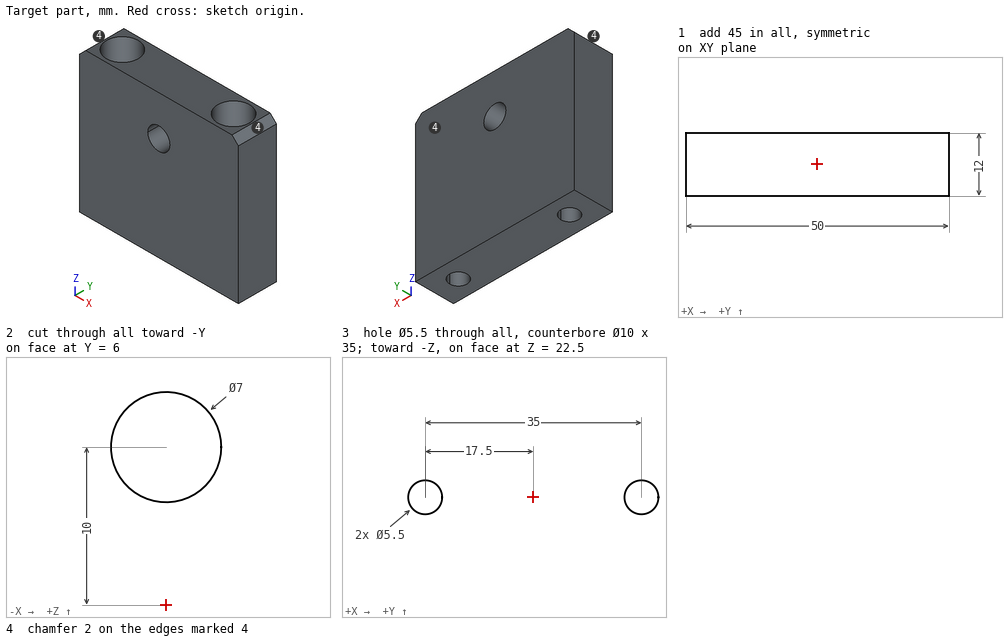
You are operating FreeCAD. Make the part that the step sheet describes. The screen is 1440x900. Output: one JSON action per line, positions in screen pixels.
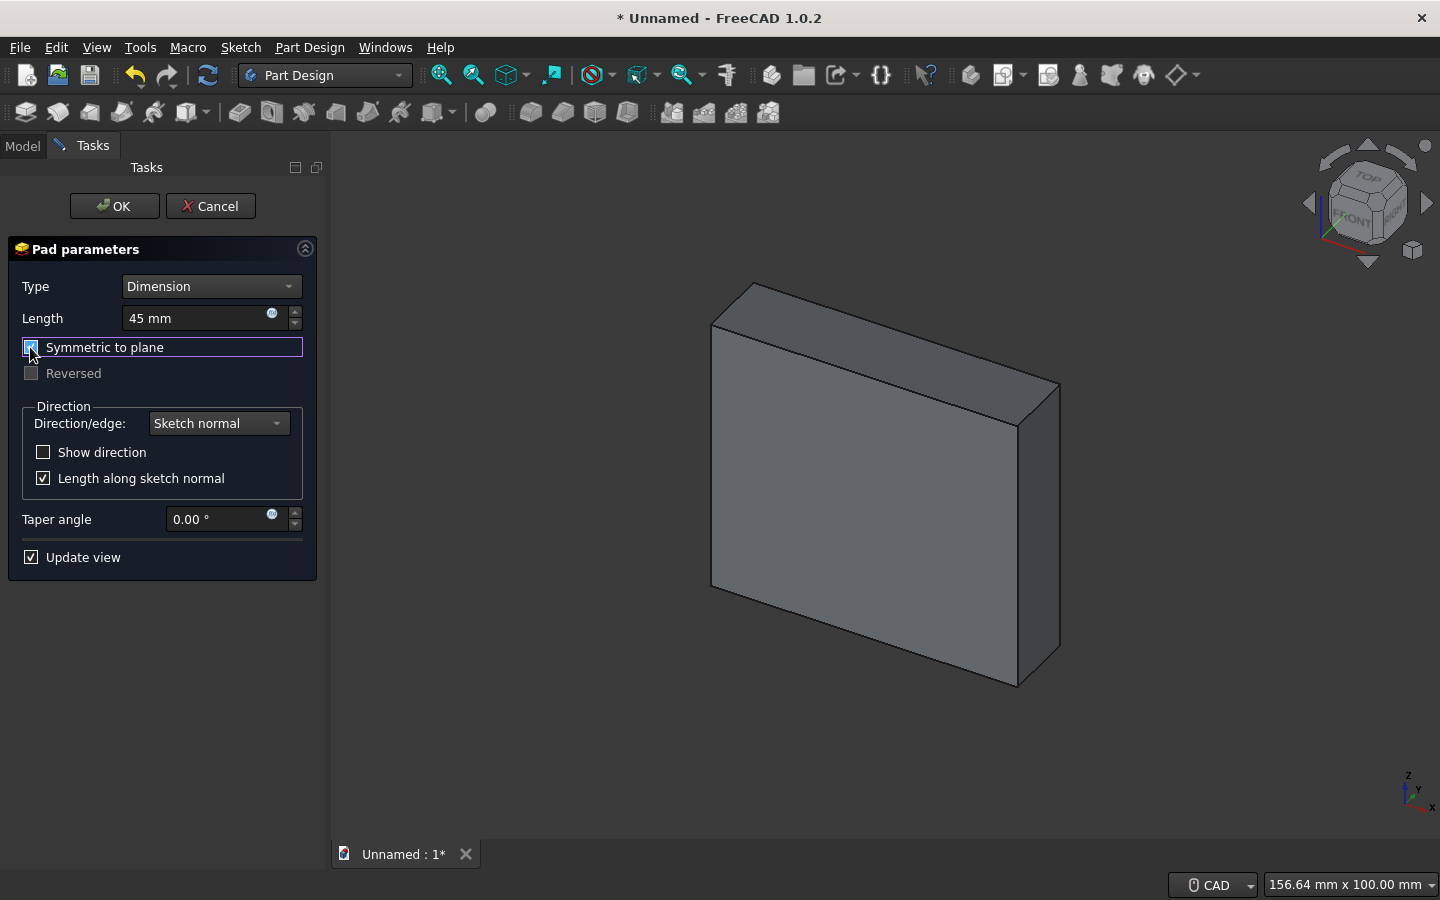
{"action": "left_click", "coordinate": [115, 206]}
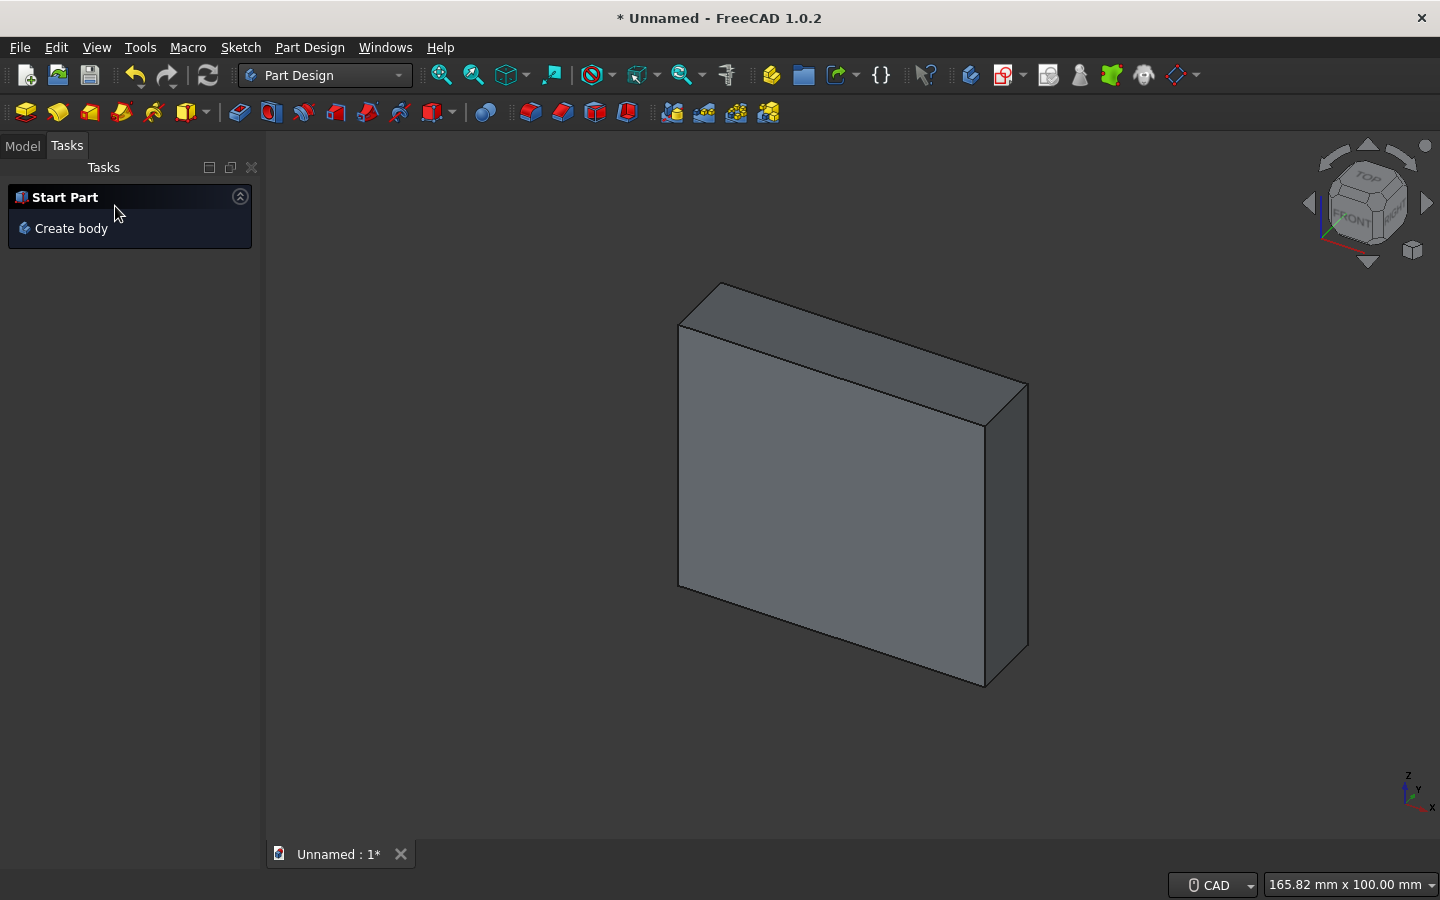
{"action": "key", "text": "4"}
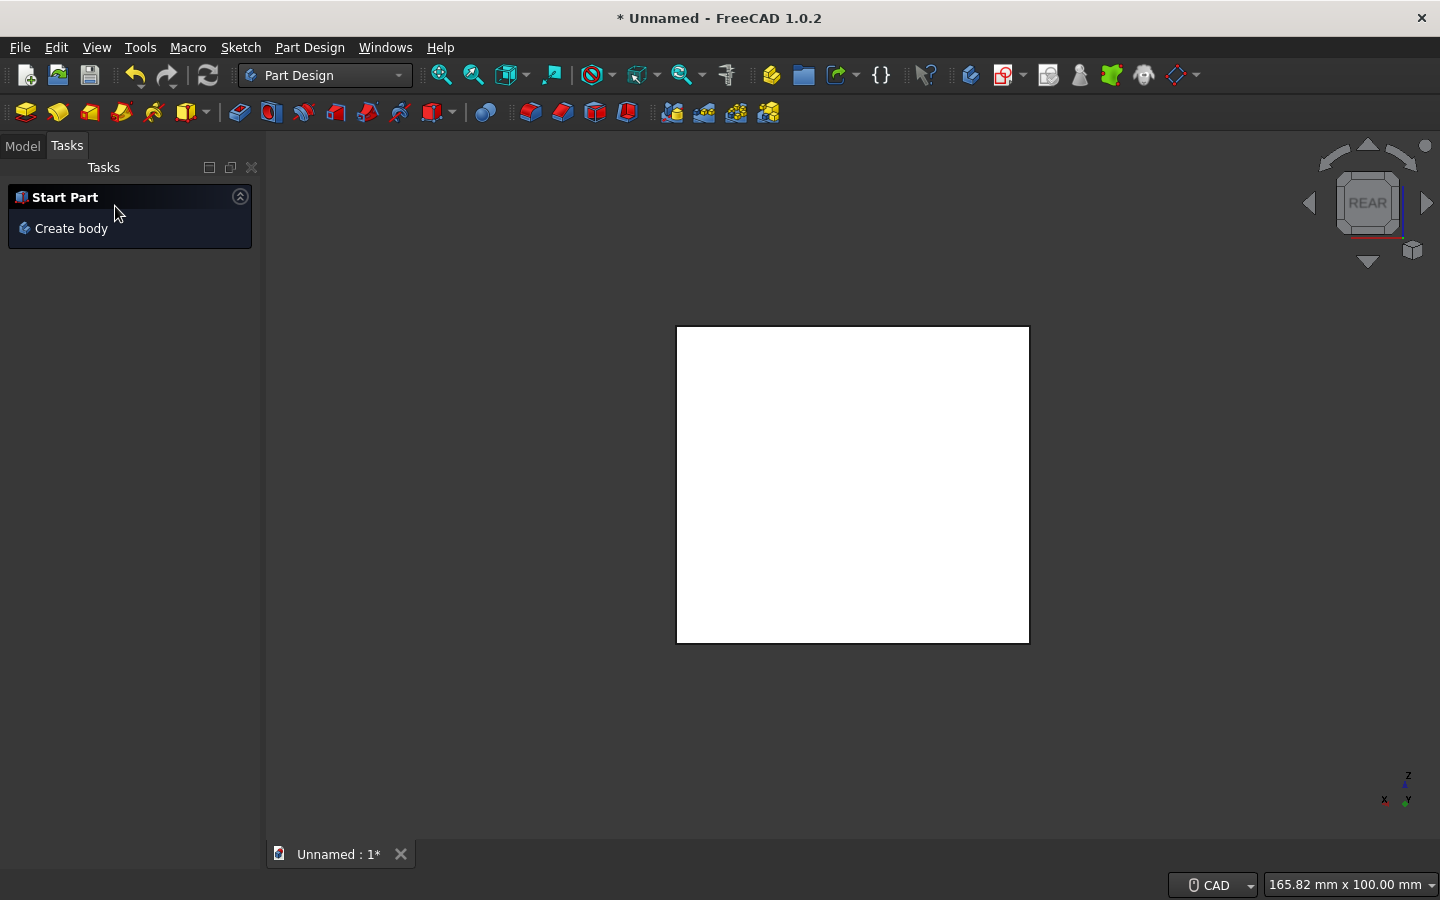
{"action": "left_click", "coordinate": [442, 76]}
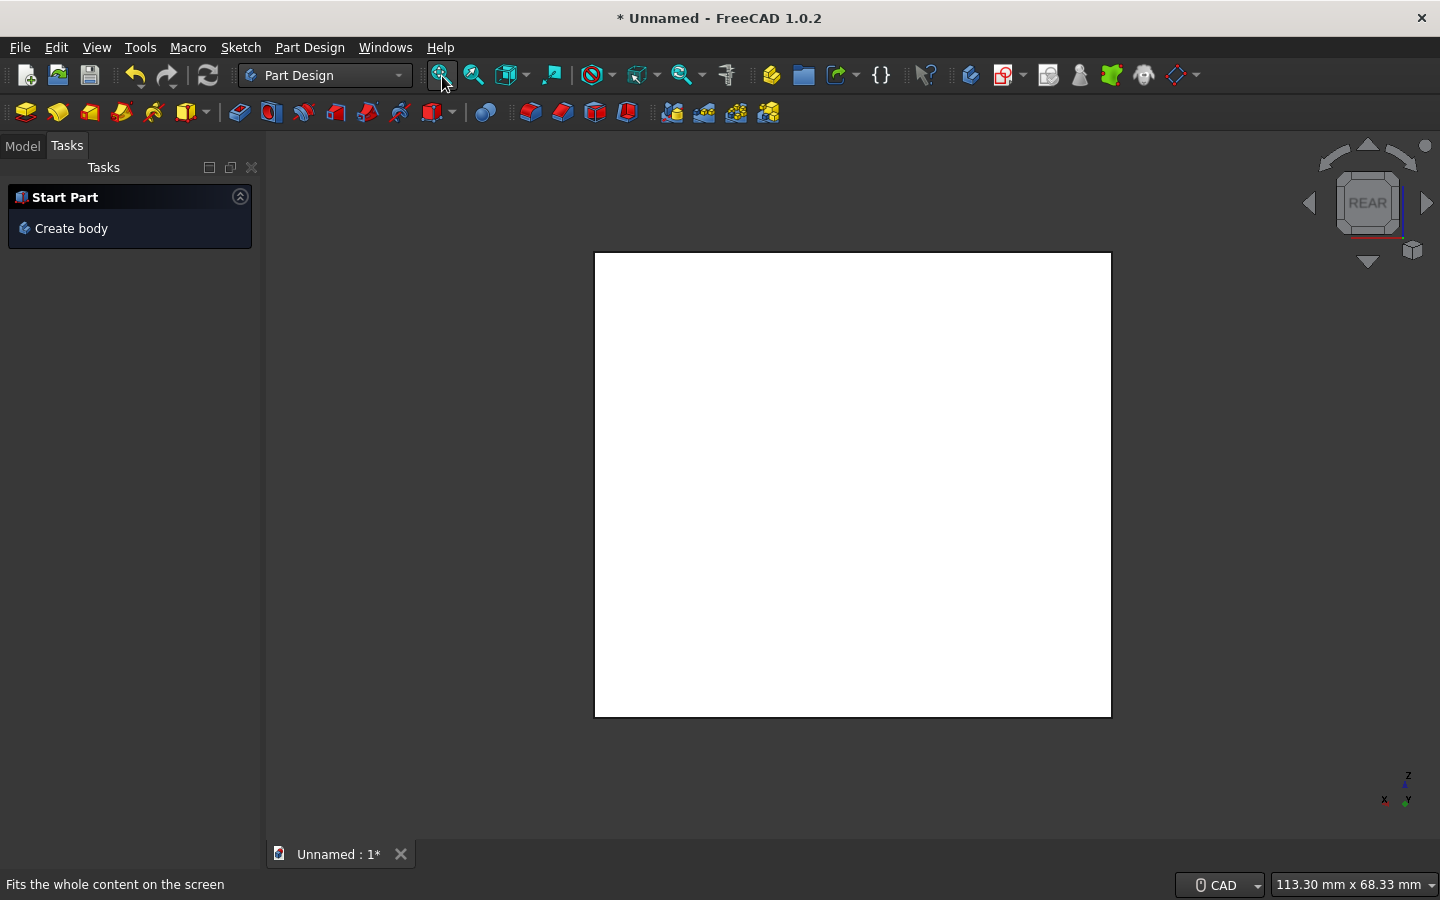
{"action": "left_click", "coordinate": [853, 484]}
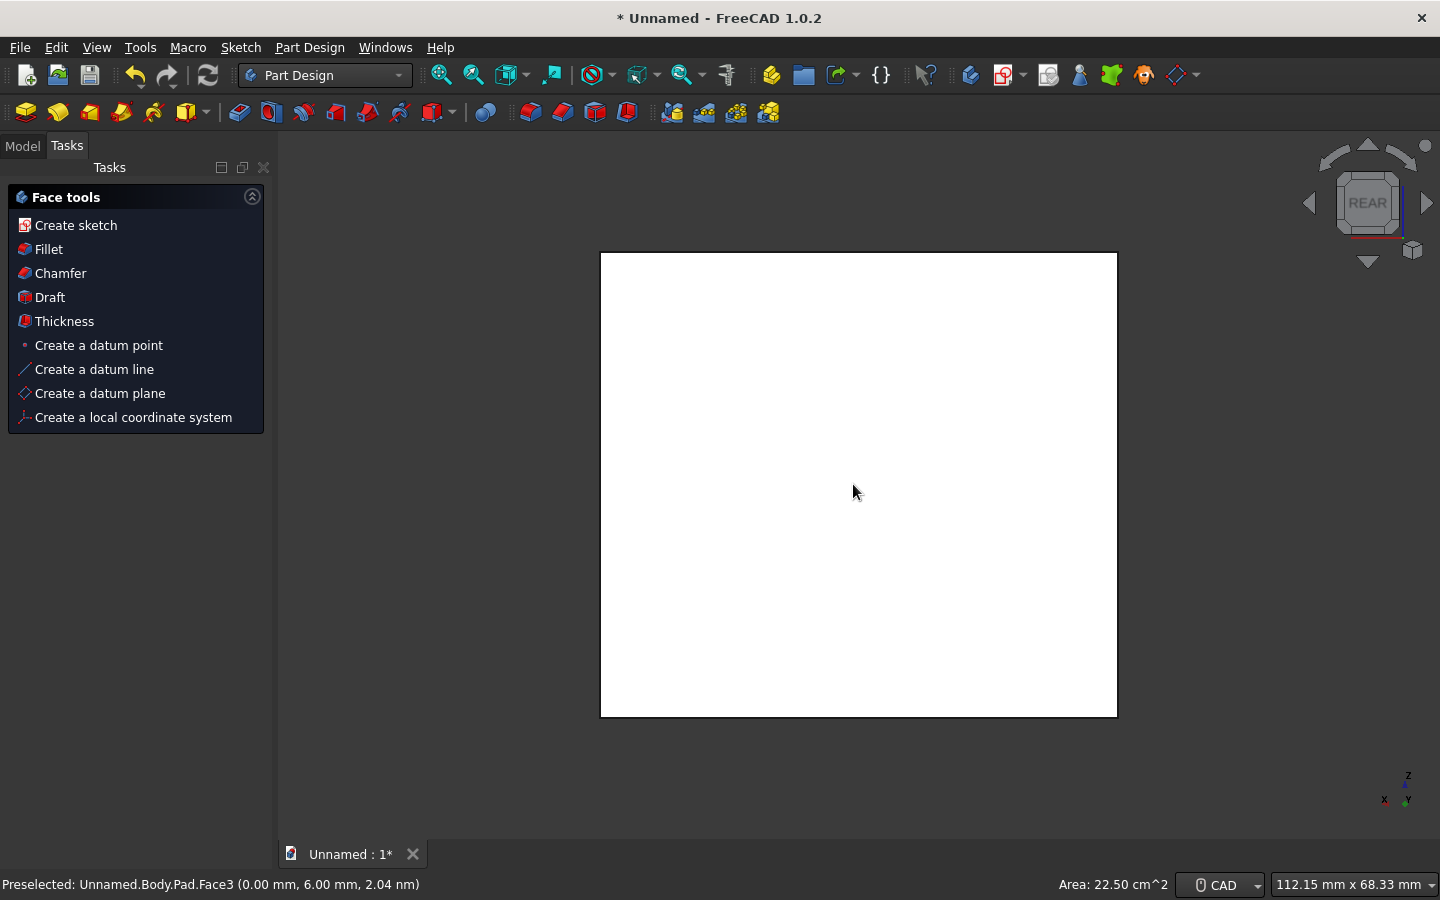
{"action": "left_click", "coordinate": [1004, 76]}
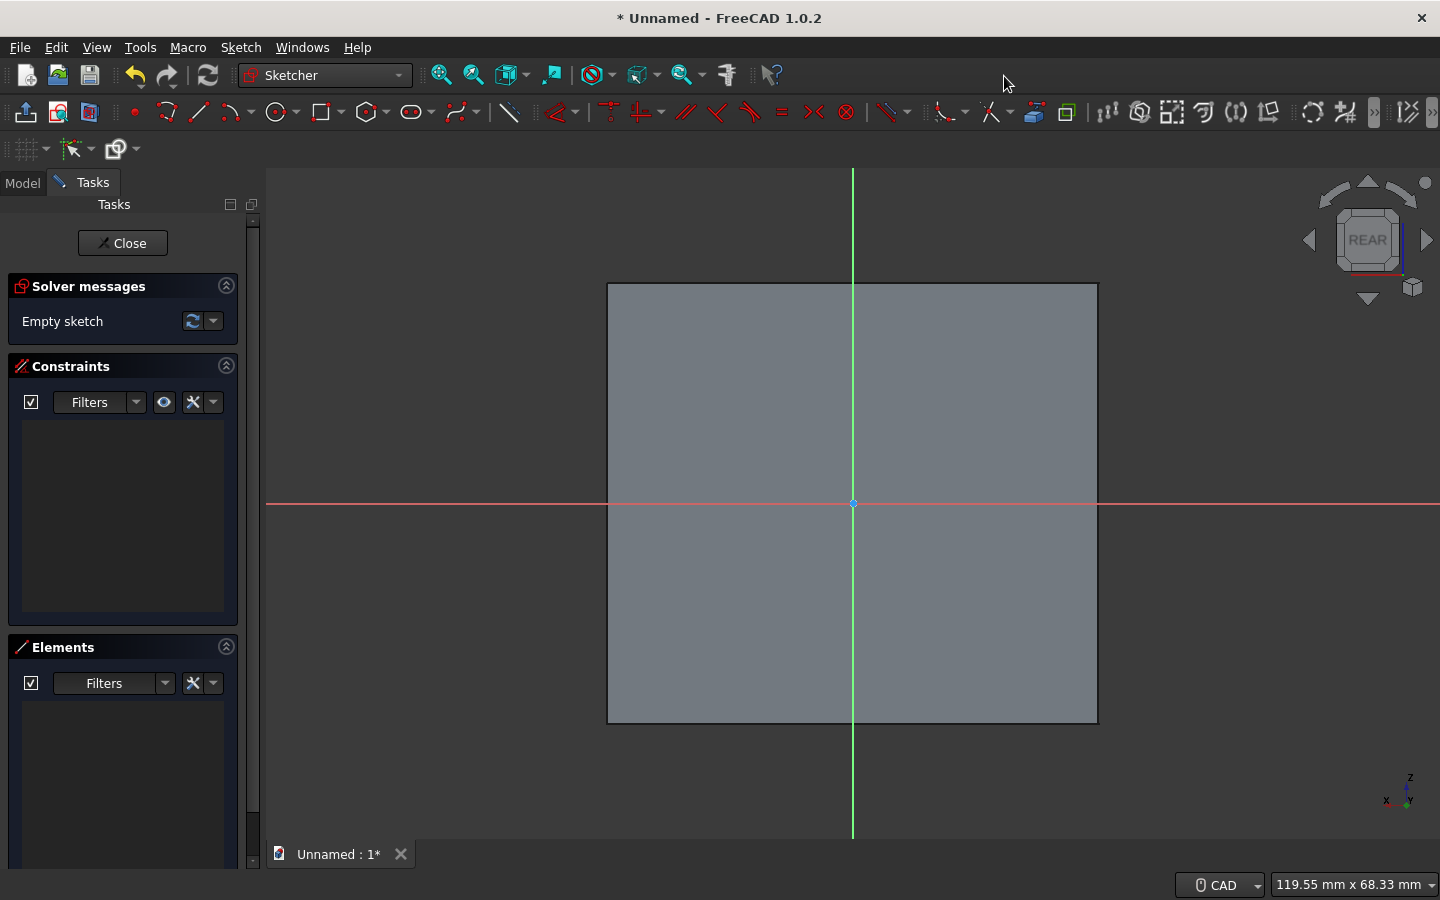
{"action": "scroll", "coordinate": [883, 409], "scroll_direction": "up", "scroll_amount": 6}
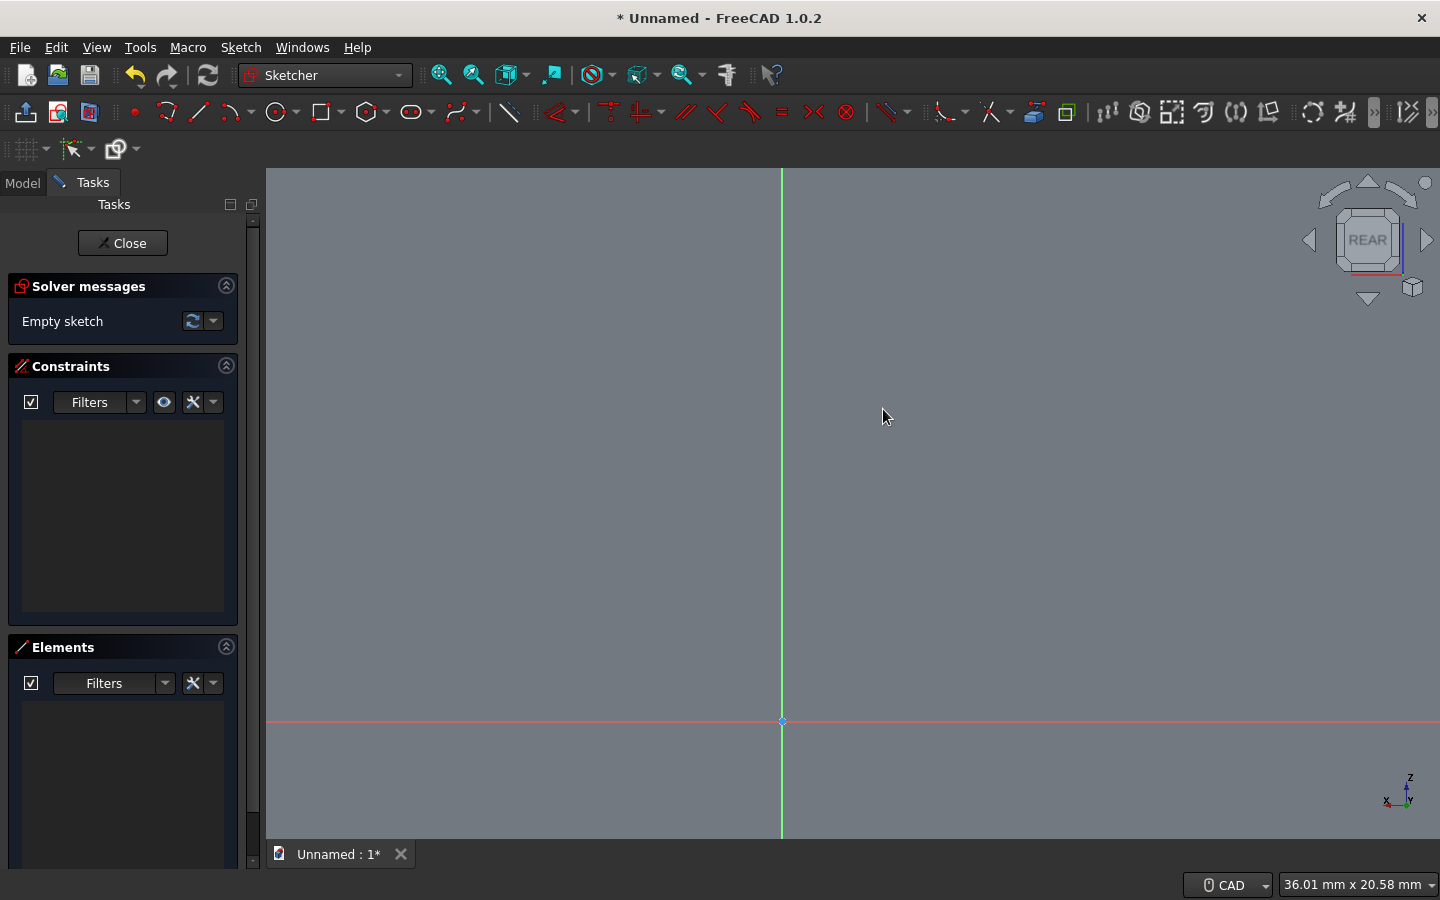
{"action": "key", "text": "g c"}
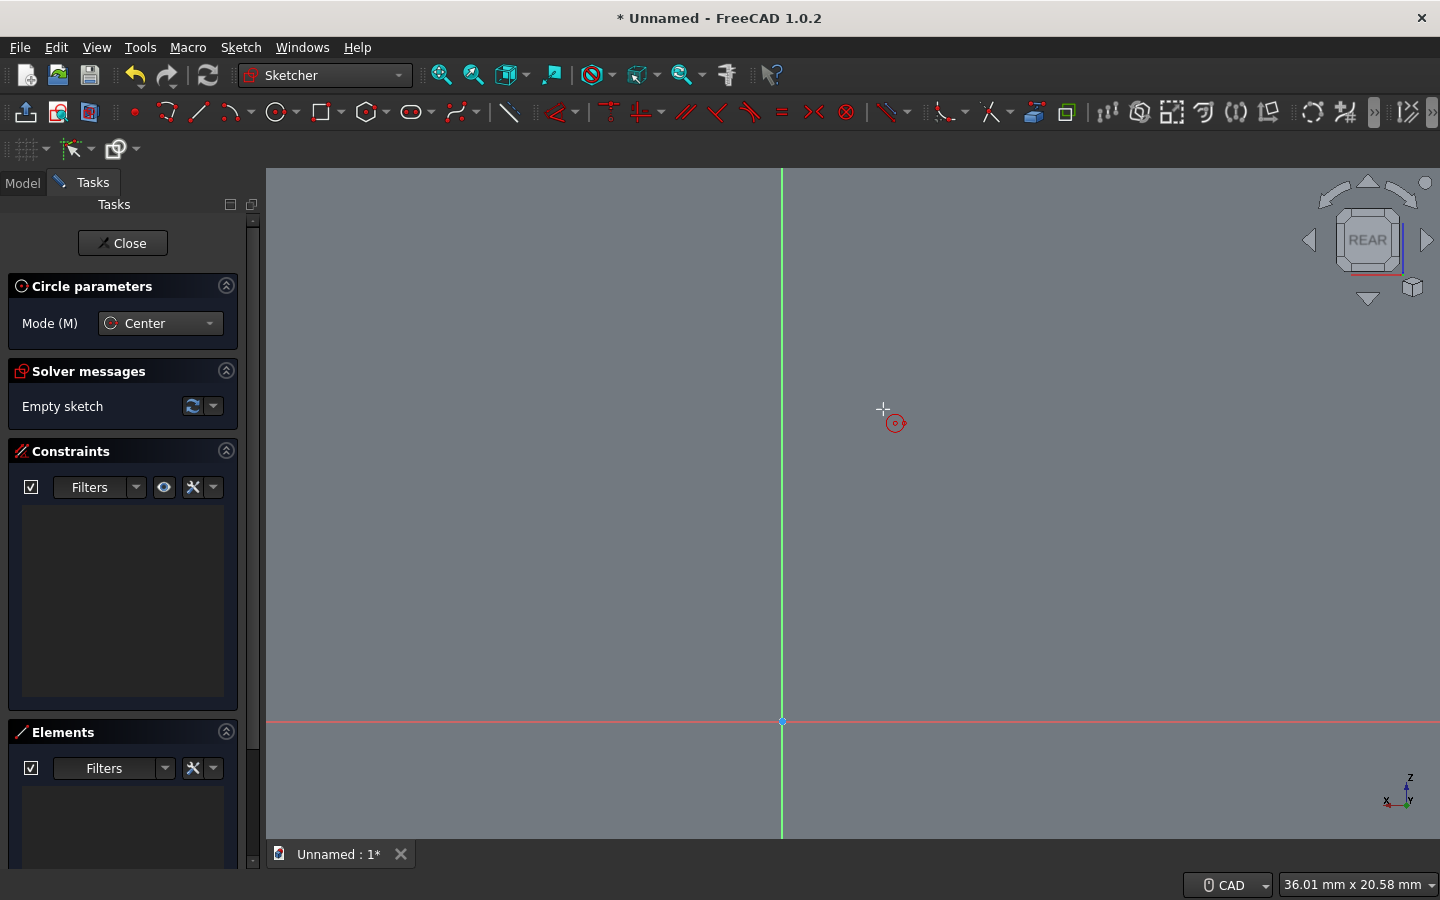
{"action": "left_click", "coordinate": [782, 396]}
{"action": "left_click", "coordinate": [863, 315]}
{"action": "key", "text": "Escape"}